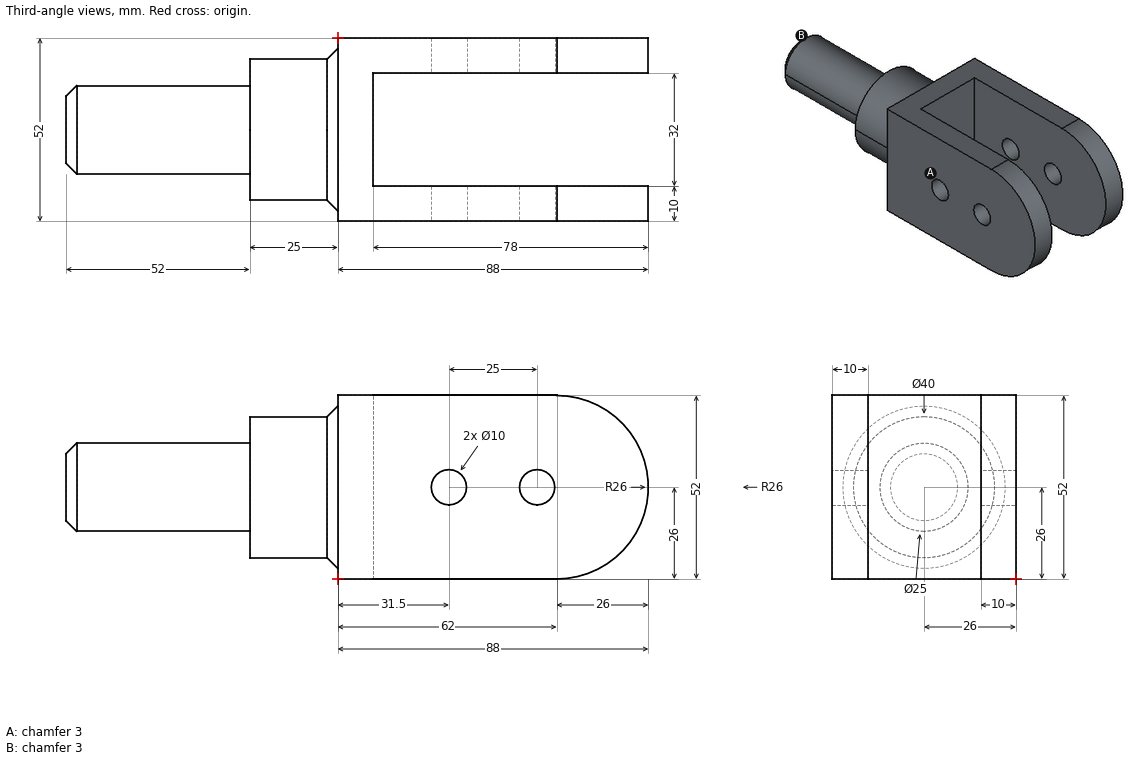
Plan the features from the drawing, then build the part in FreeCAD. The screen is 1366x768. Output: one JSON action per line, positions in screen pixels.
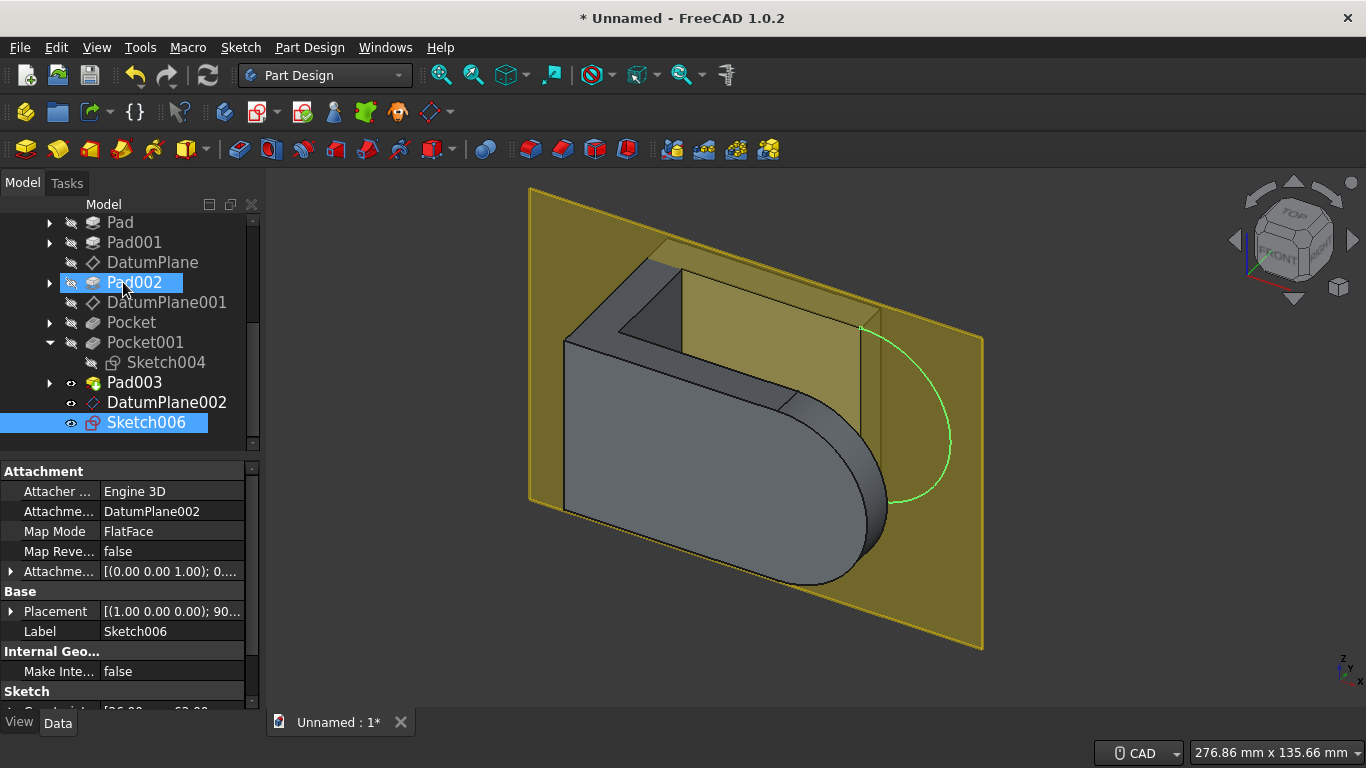
{"action": "left_click", "coordinate": [26, 150]}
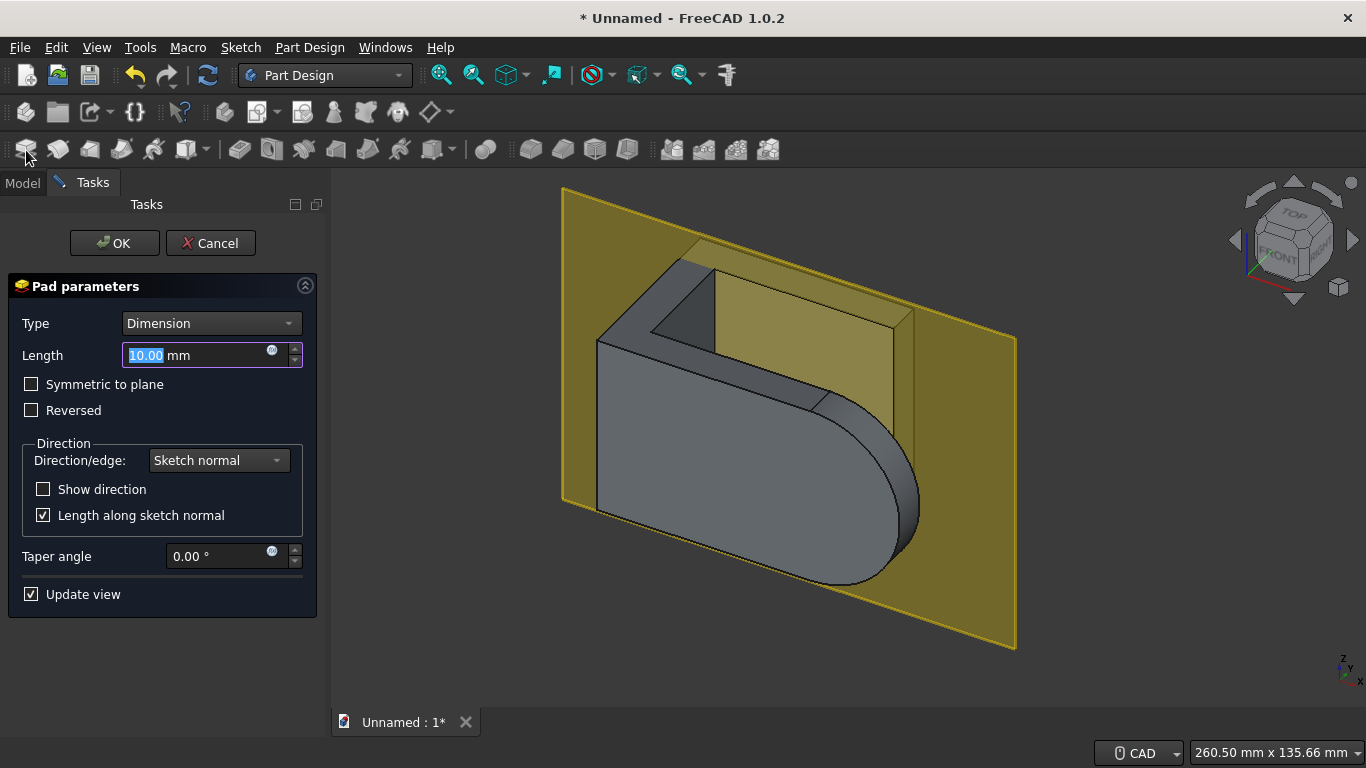
{"action": "type", "text": "10"}
{"action": "key", "text": "Tab"}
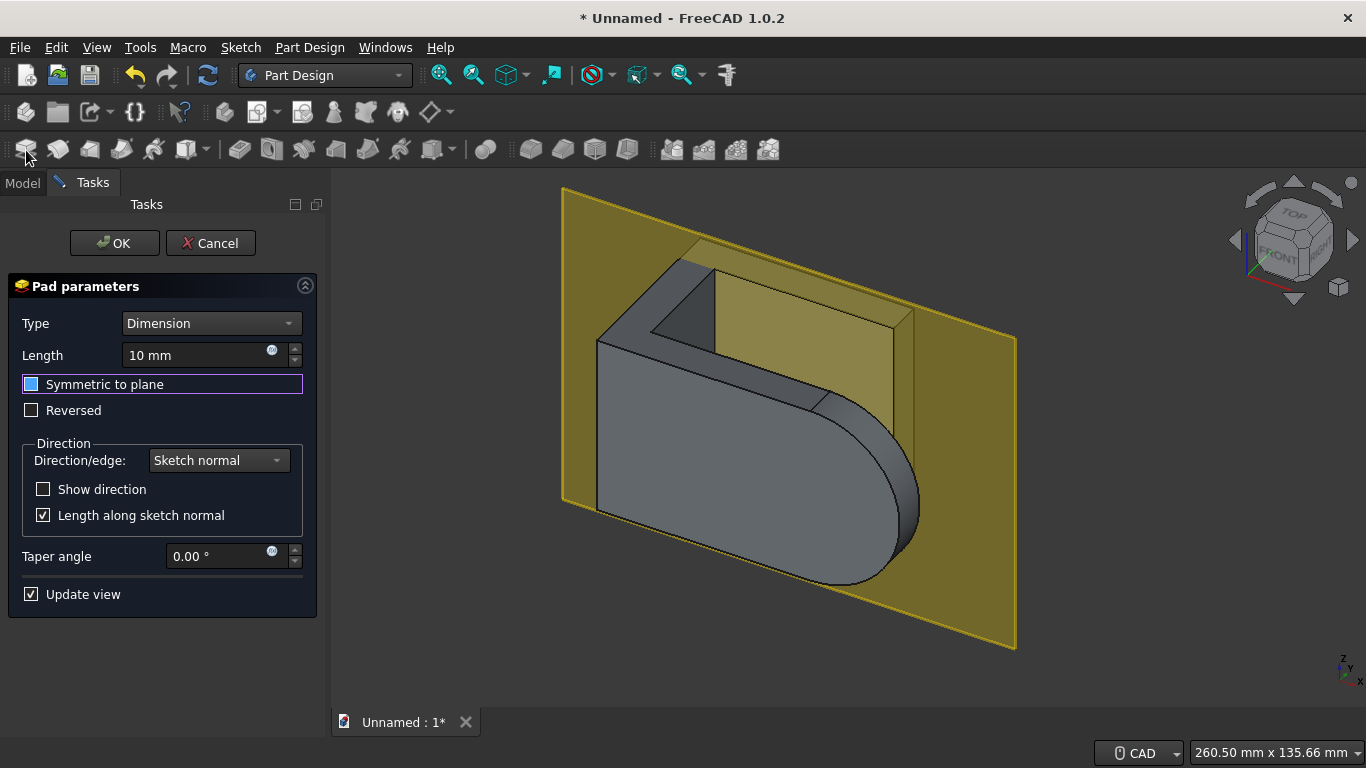
{"action": "left_click", "coordinate": [30, 410]}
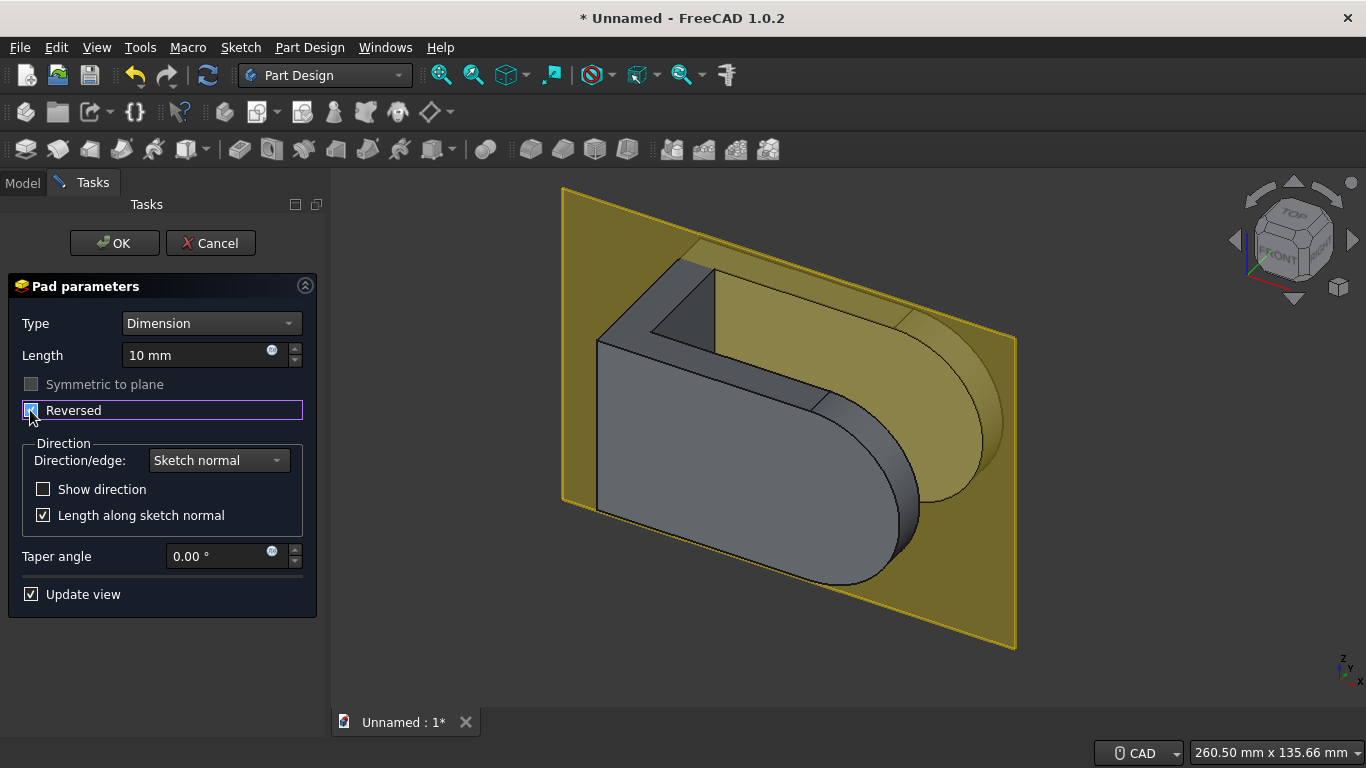
{"action": "left_click", "coordinate": [115, 243]}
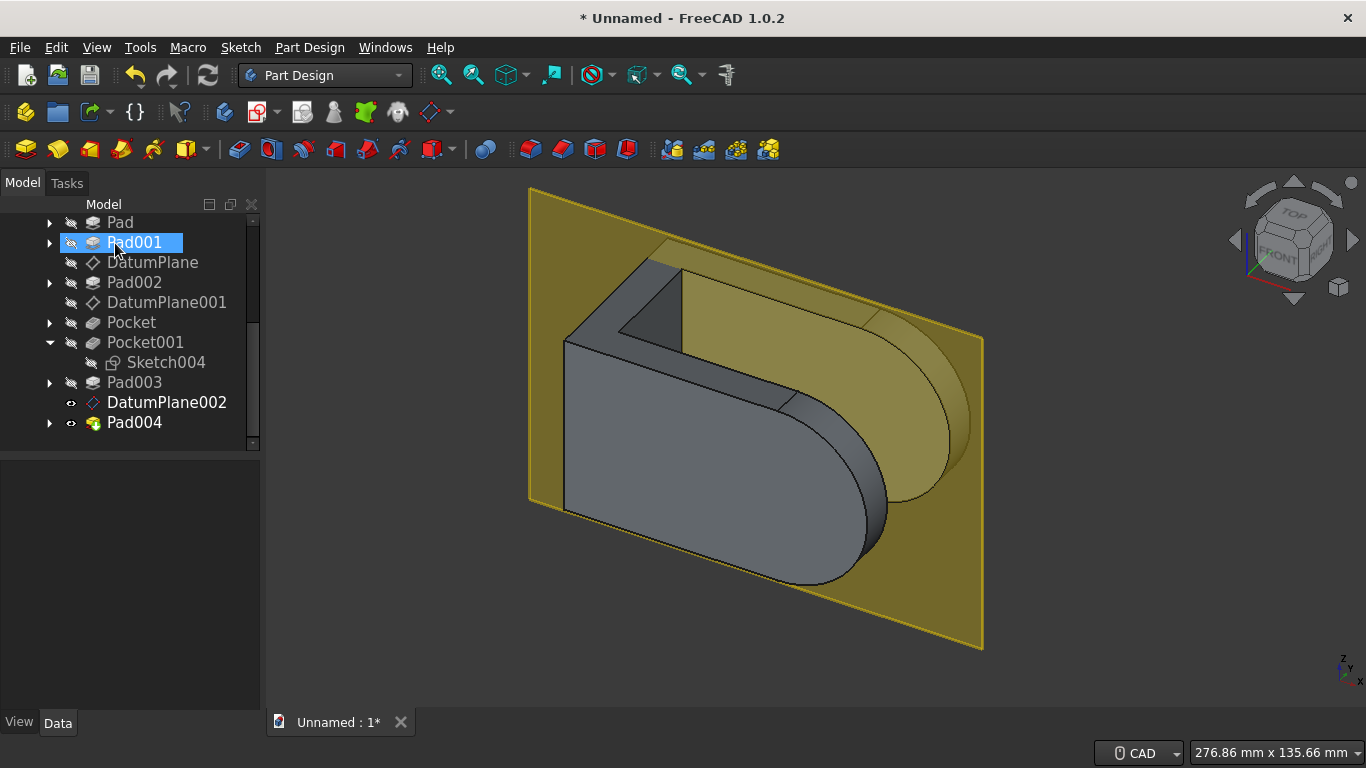
{"action": "left_click", "coordinate": [116, 403]}
{"action": "key", "text": "space"}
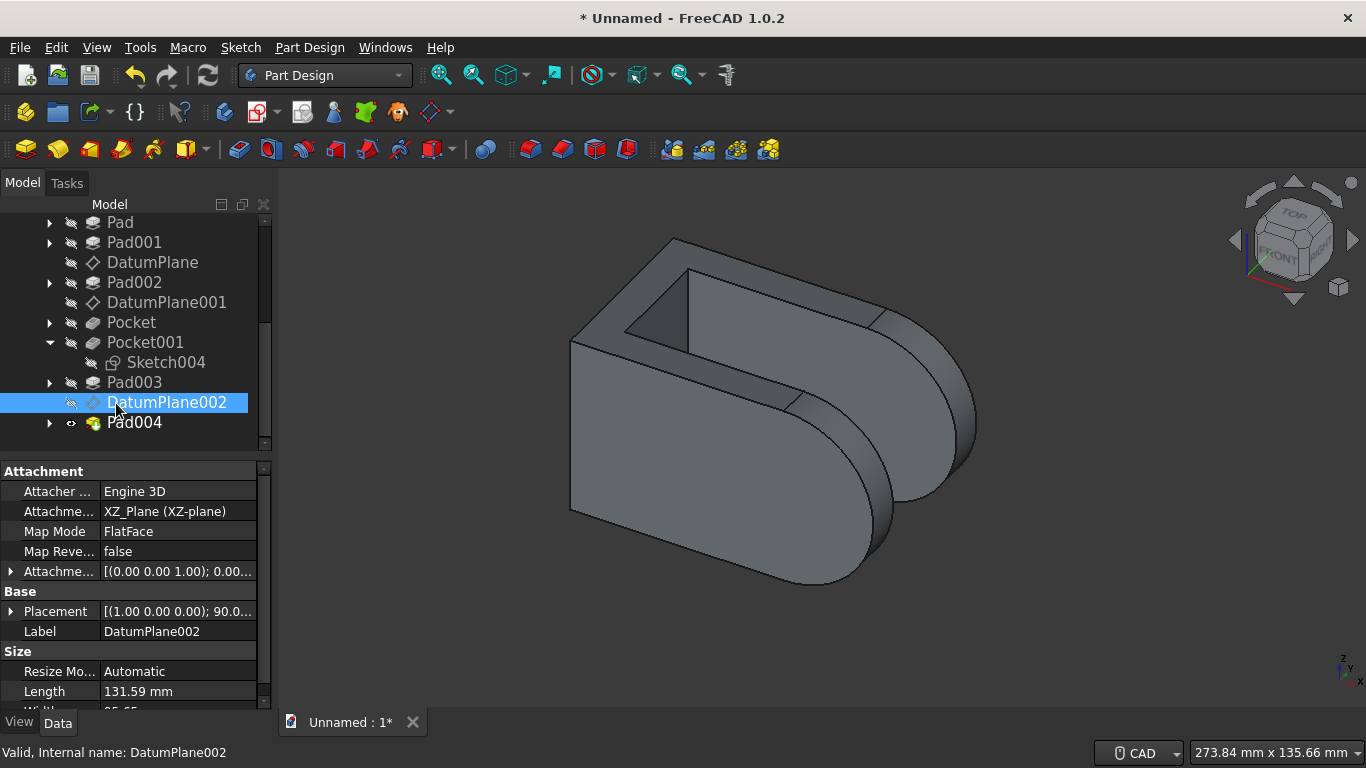
{"action": "key", "text": "6"}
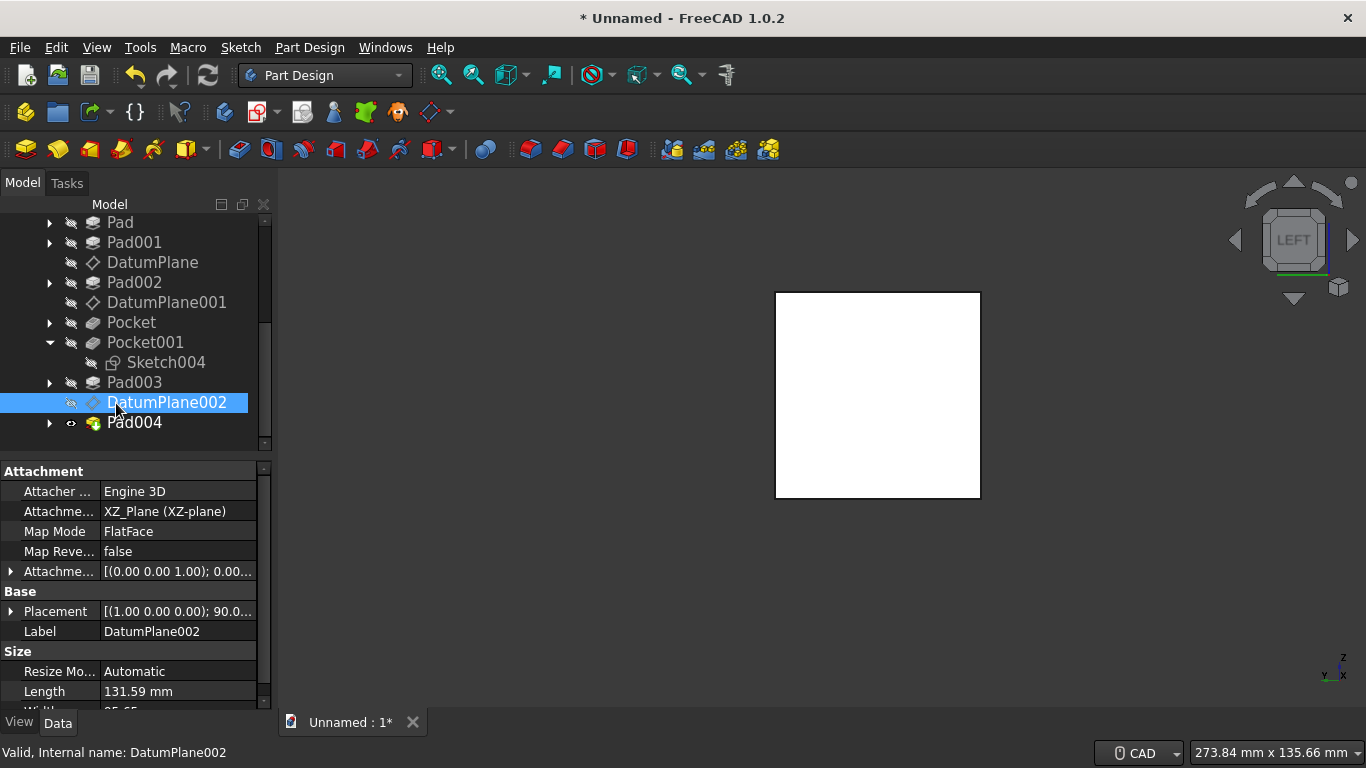
{"action": "left_click", "coordinate": [442, 76]}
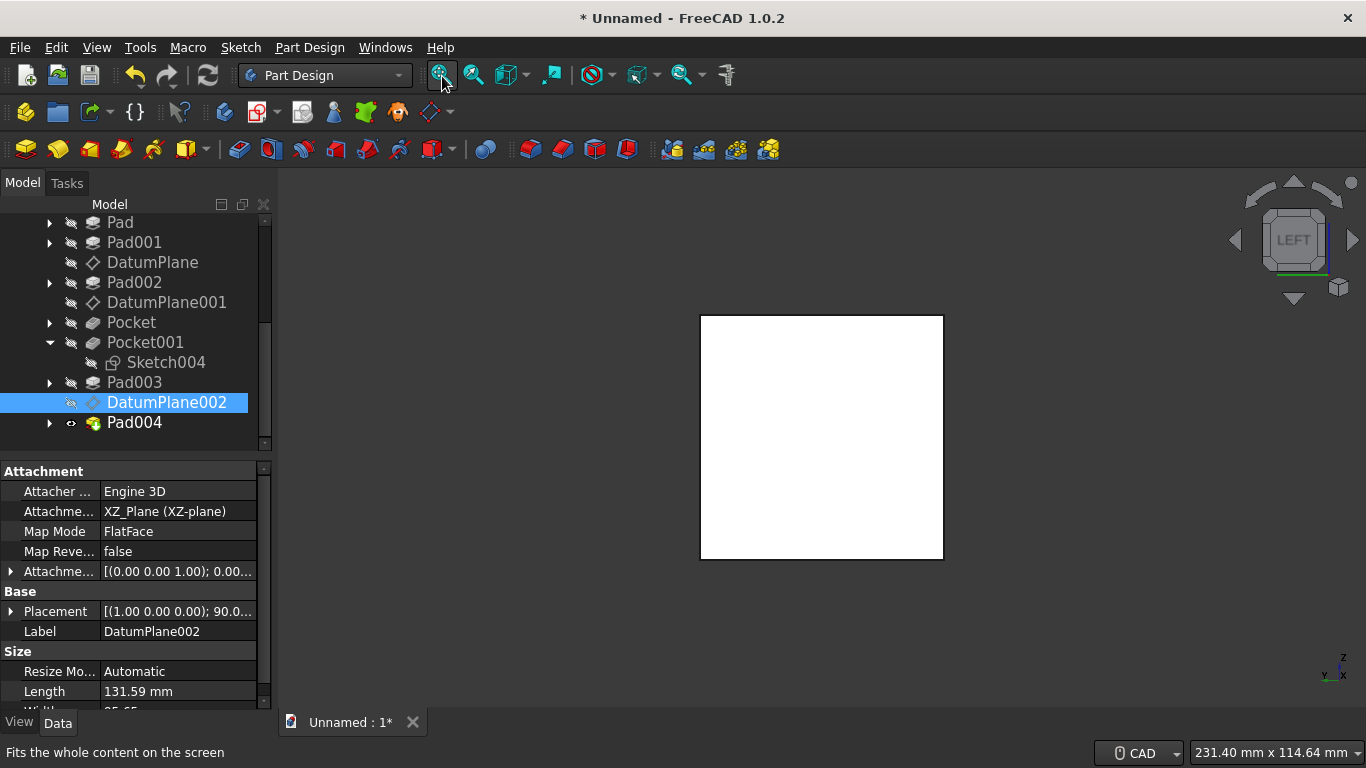
{"action": "left_click", "coordinate": [822, 436]}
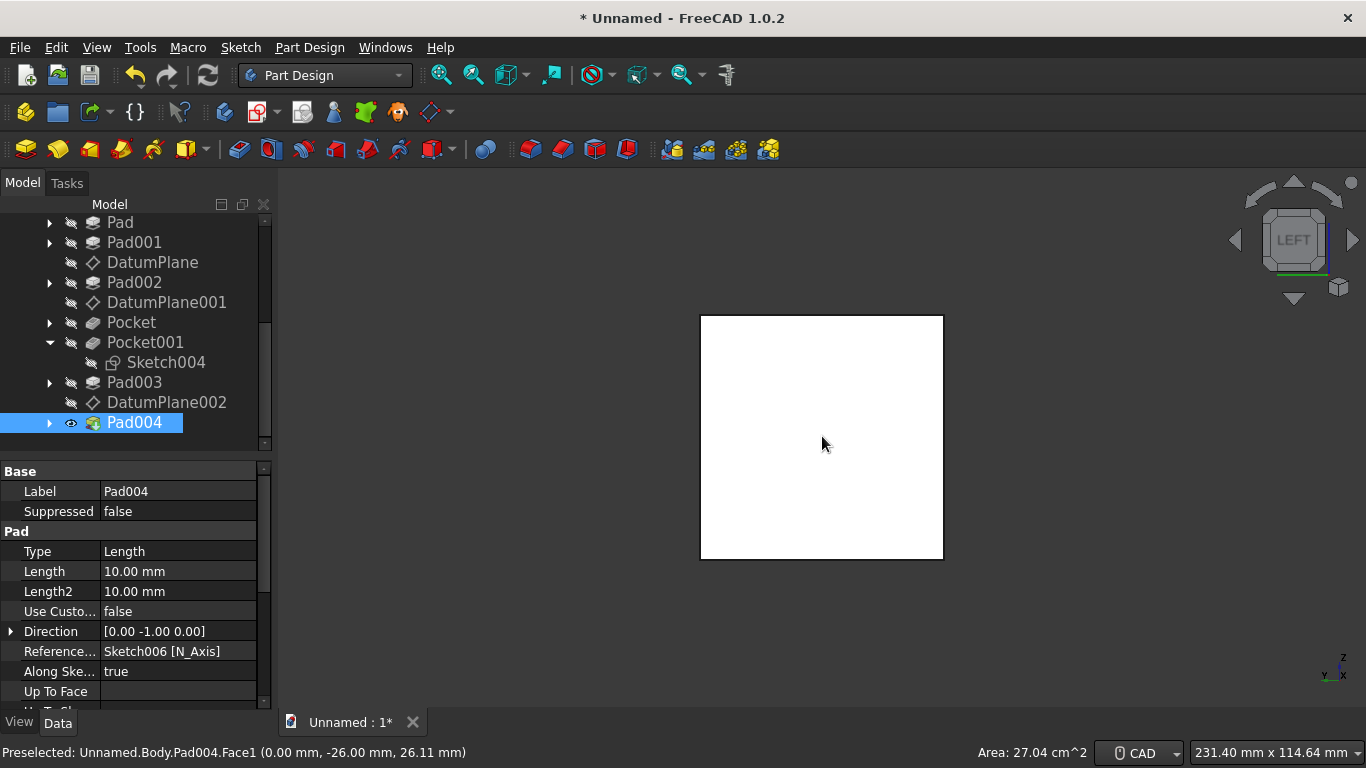
{"action": "left_click", "coordinate": [258, 112]}